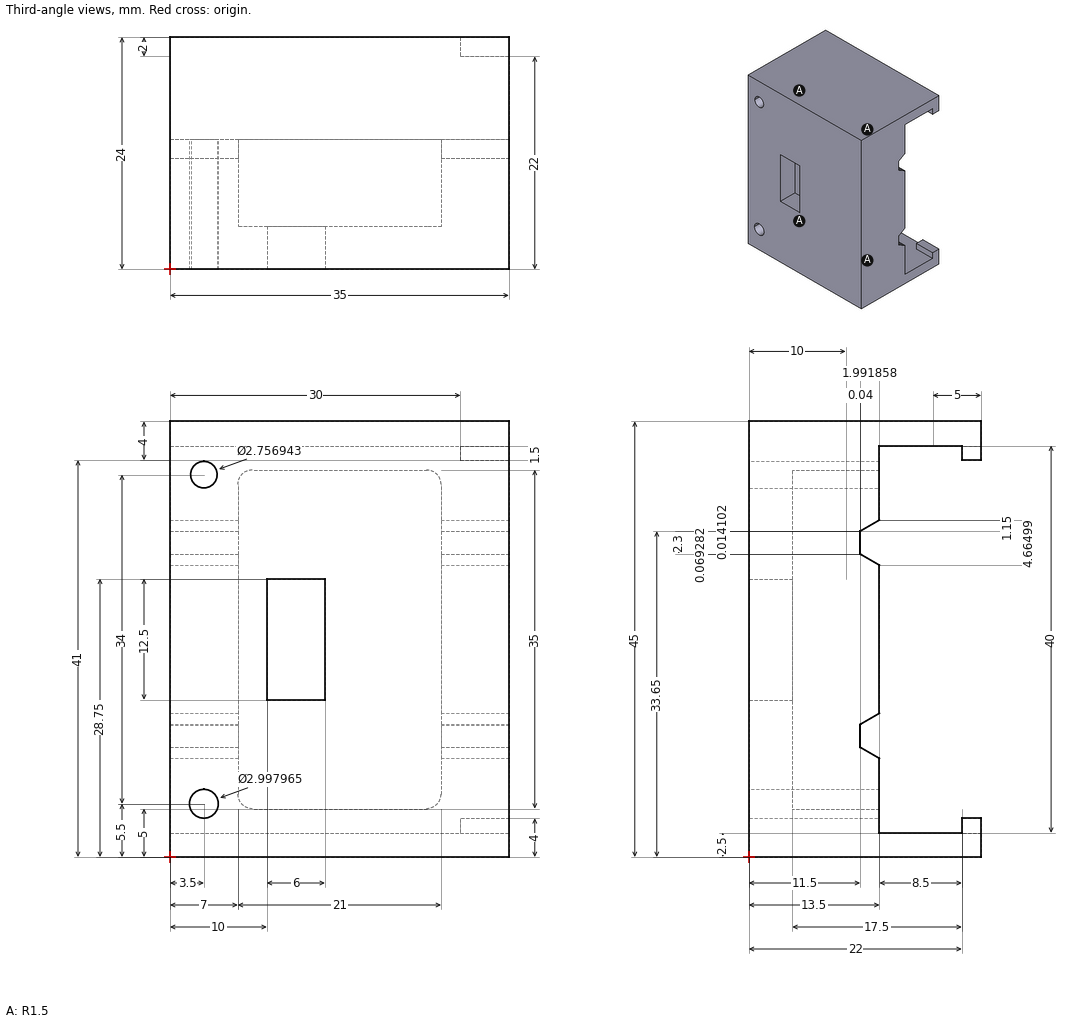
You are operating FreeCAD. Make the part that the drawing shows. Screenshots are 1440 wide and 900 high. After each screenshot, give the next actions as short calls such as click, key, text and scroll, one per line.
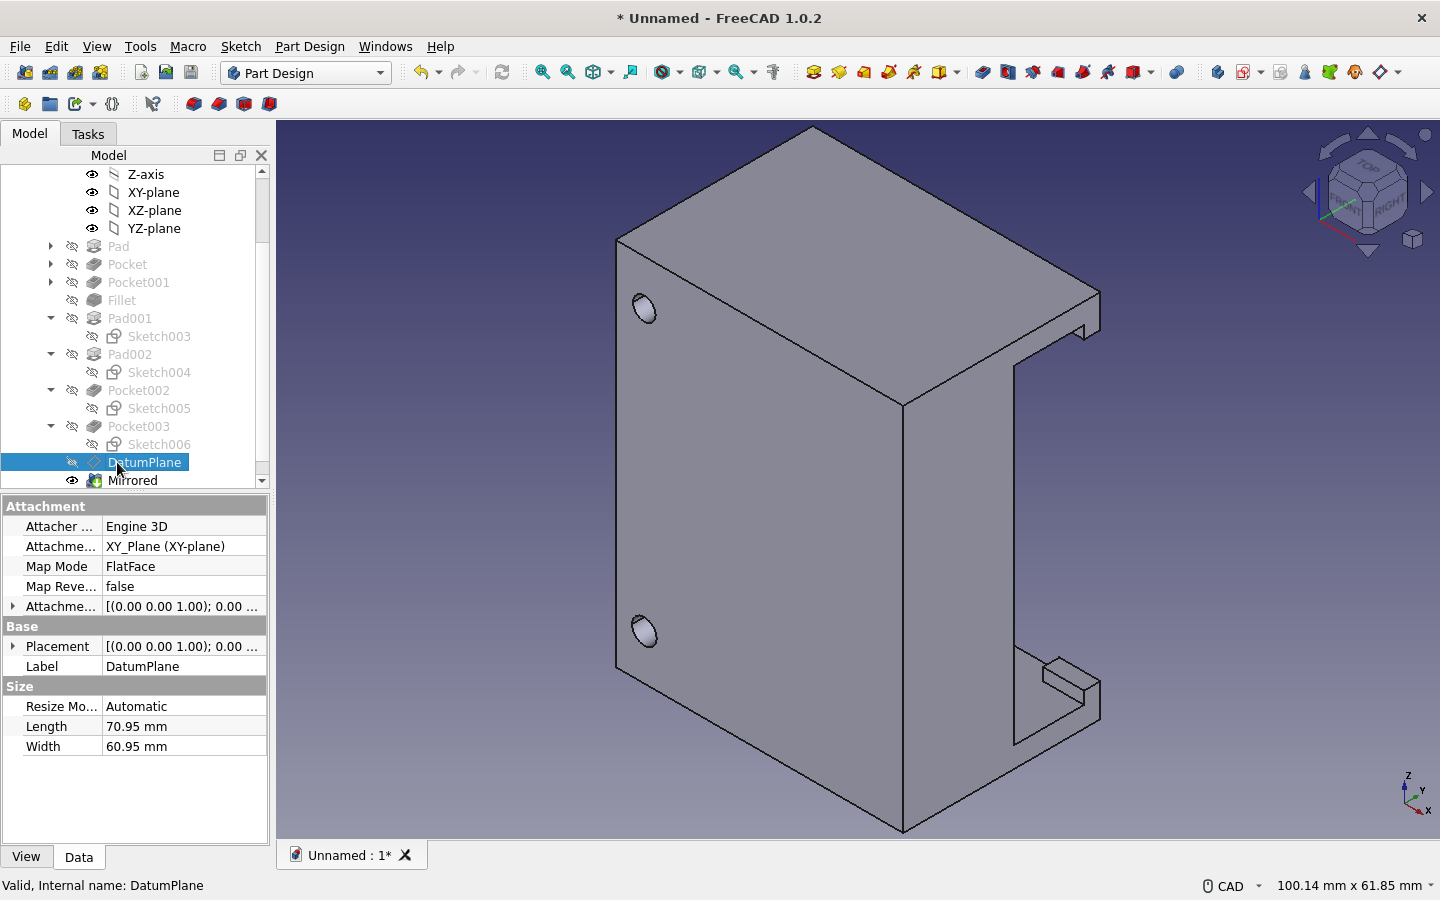
click(759, 535)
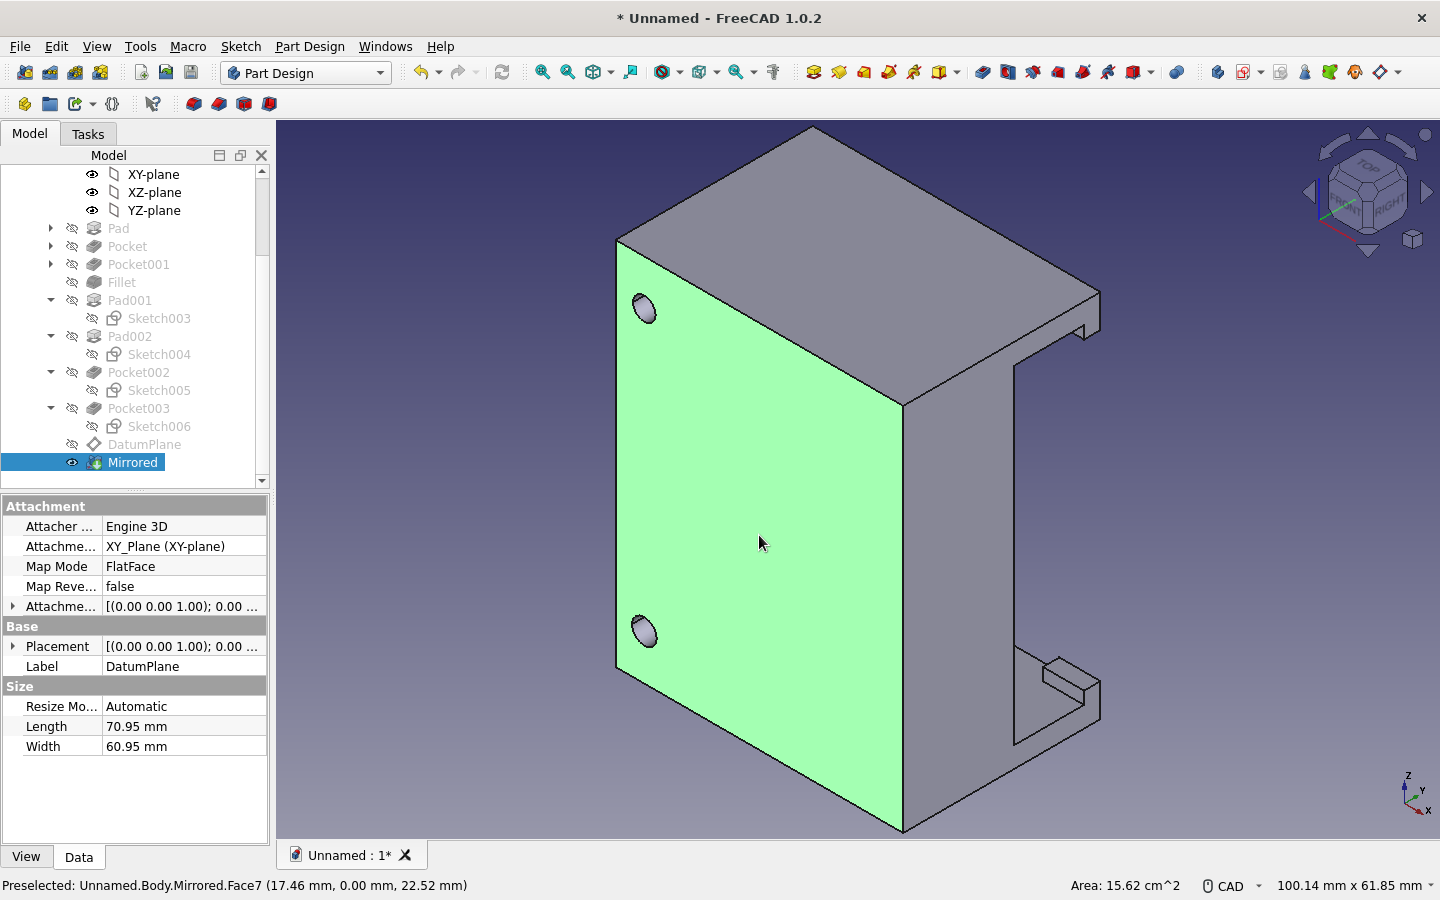
click(1242, 72)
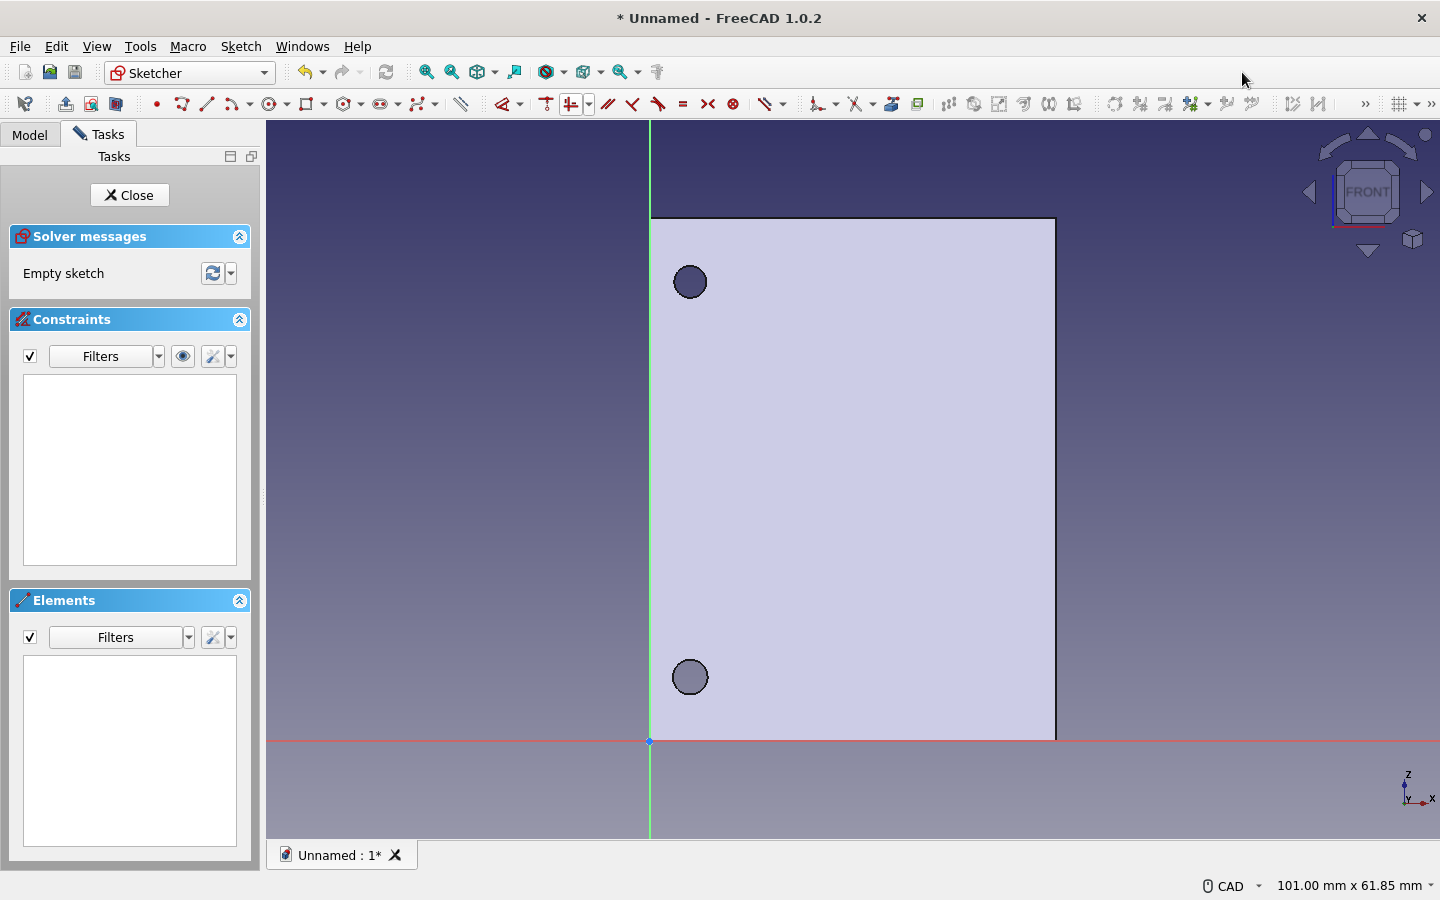
scroll(657, 766, up, 2)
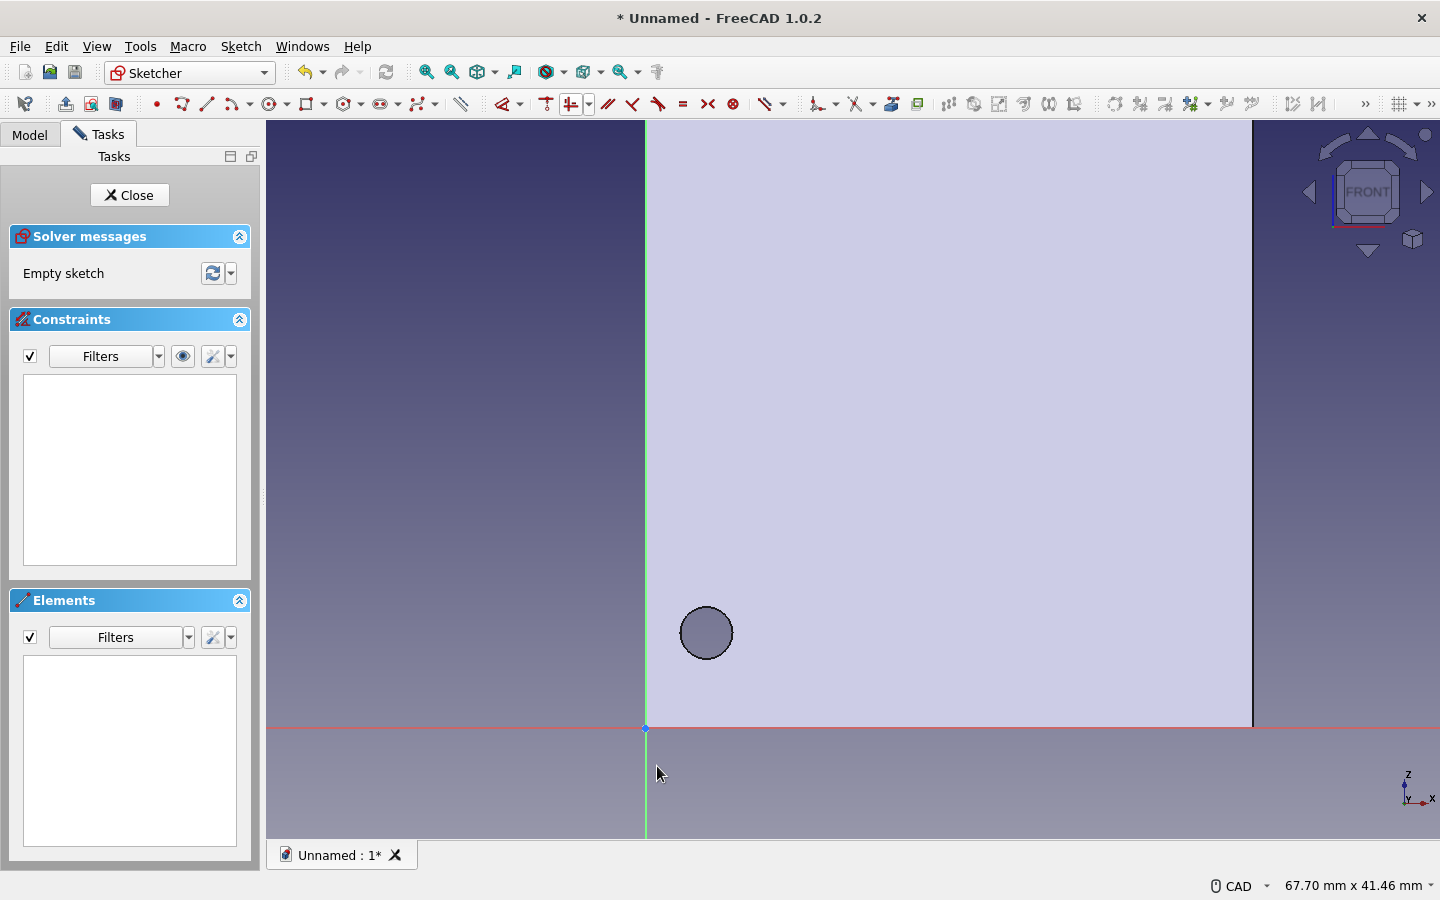
key(g)
key(r)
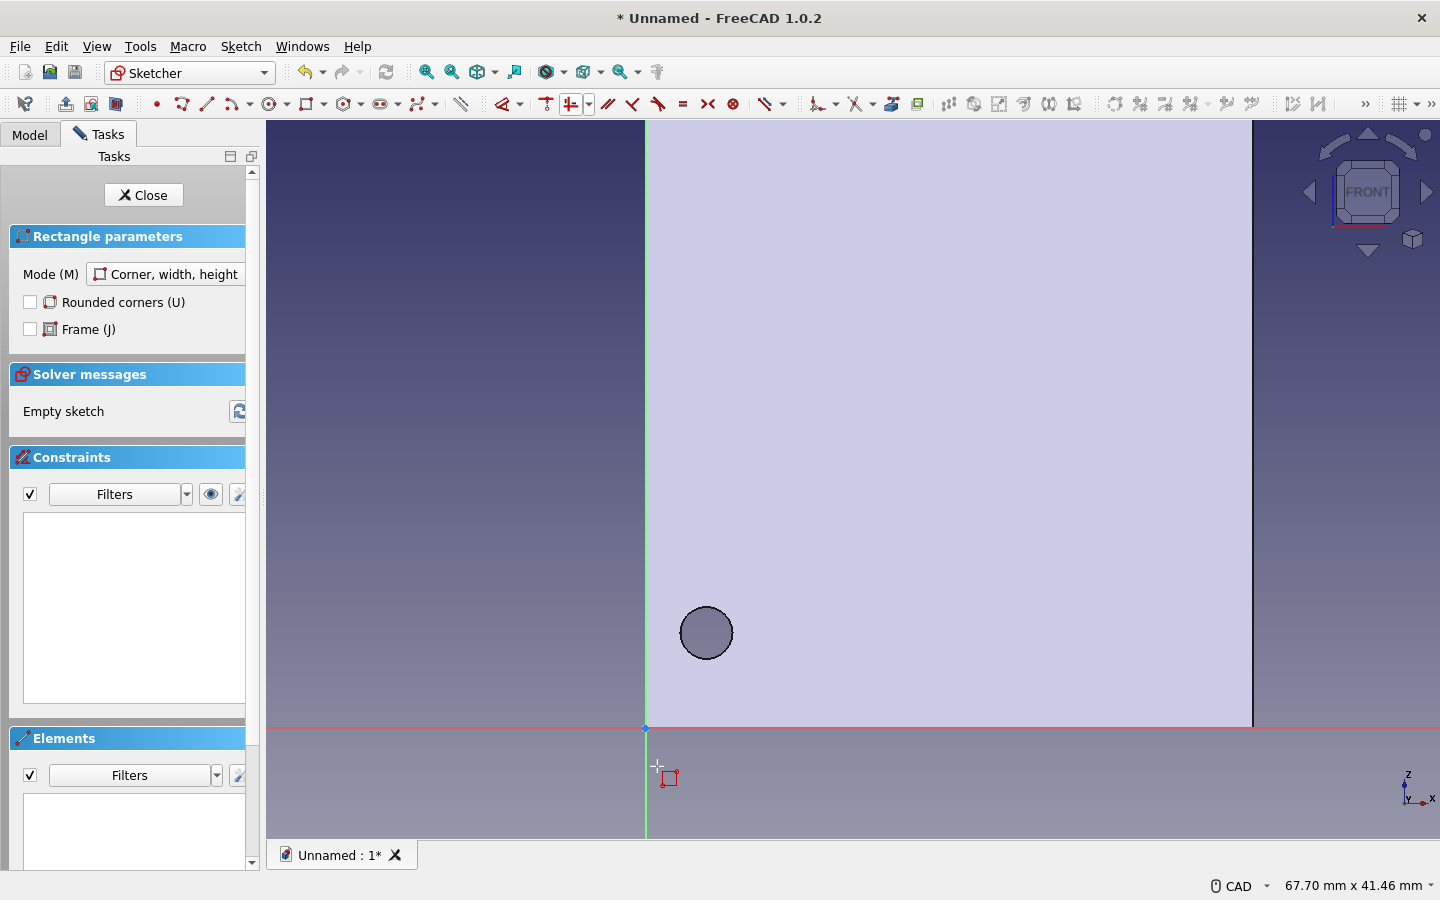
click(819, 230)
click(923, 447)
key(Escape)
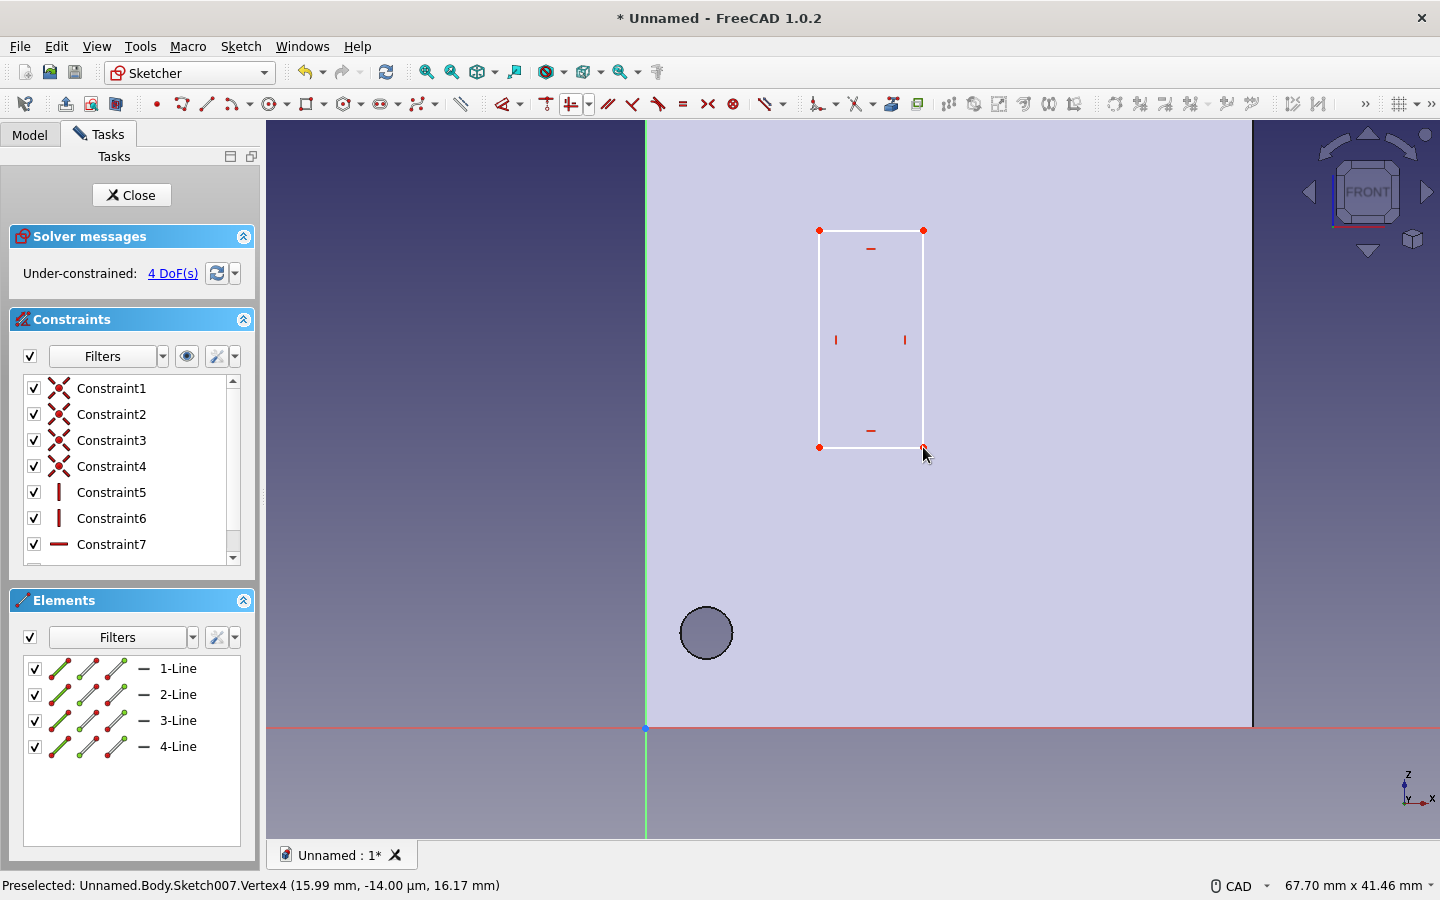
click(502, 104)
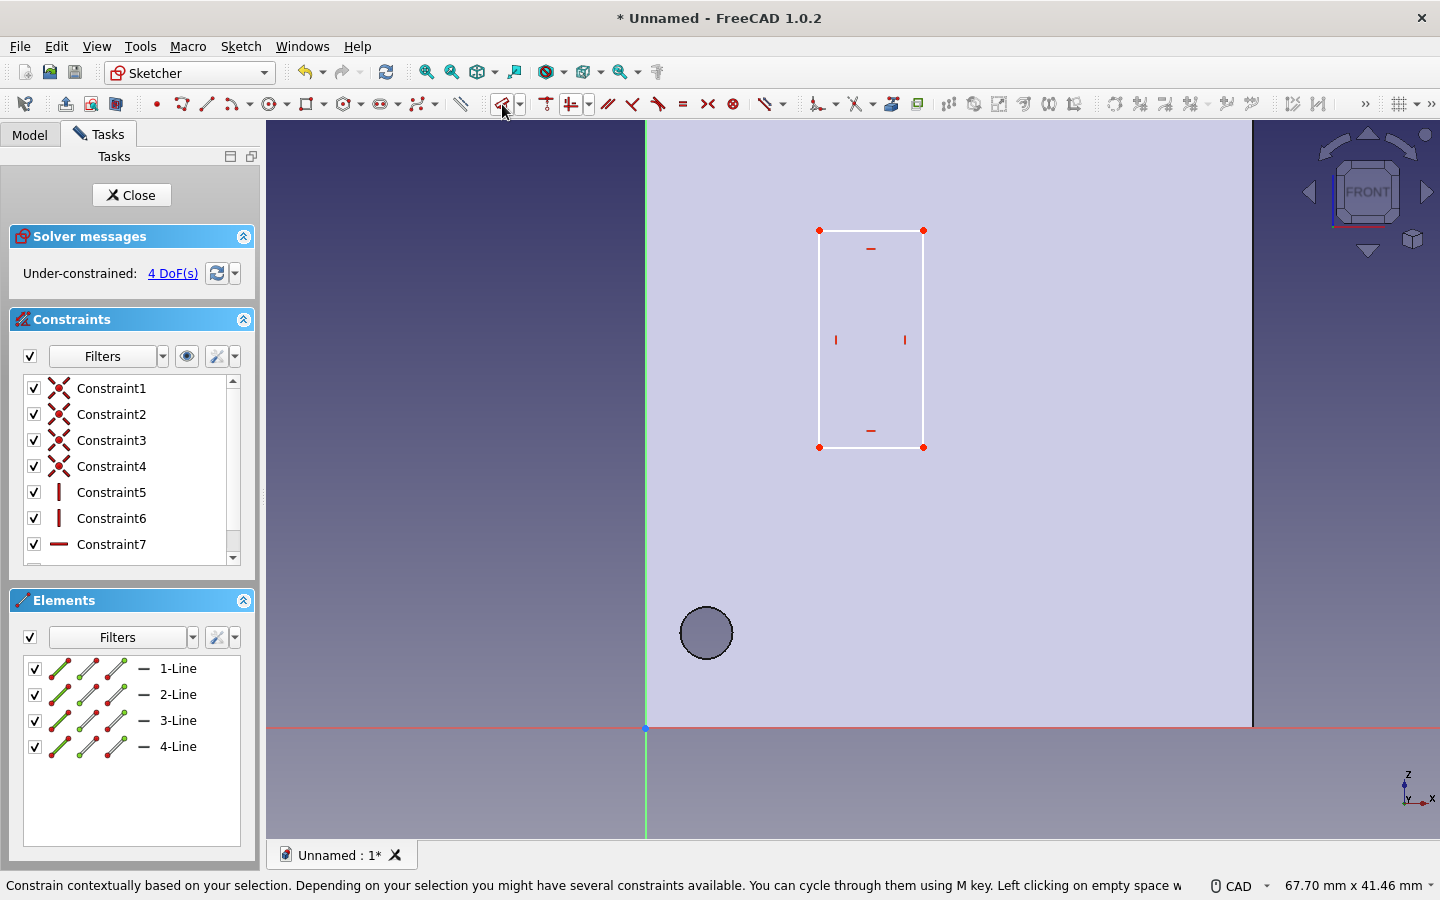
click(850, 448)
click(871, 414)